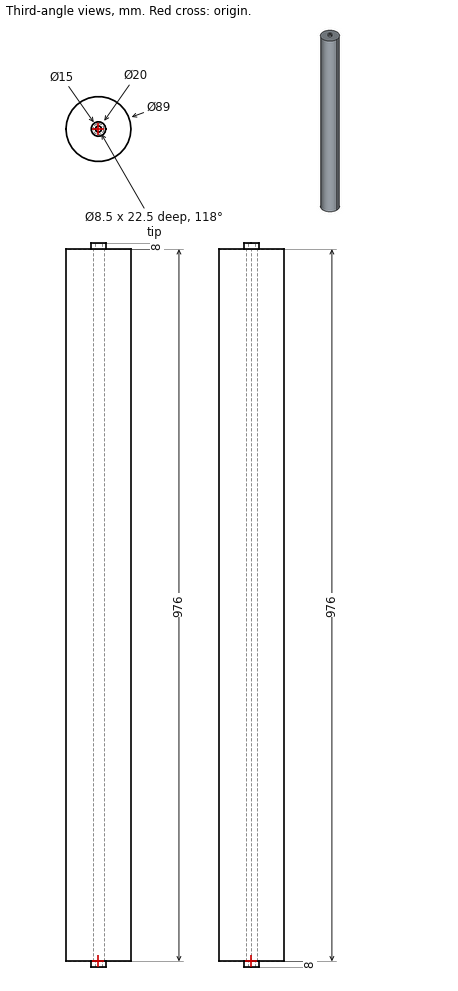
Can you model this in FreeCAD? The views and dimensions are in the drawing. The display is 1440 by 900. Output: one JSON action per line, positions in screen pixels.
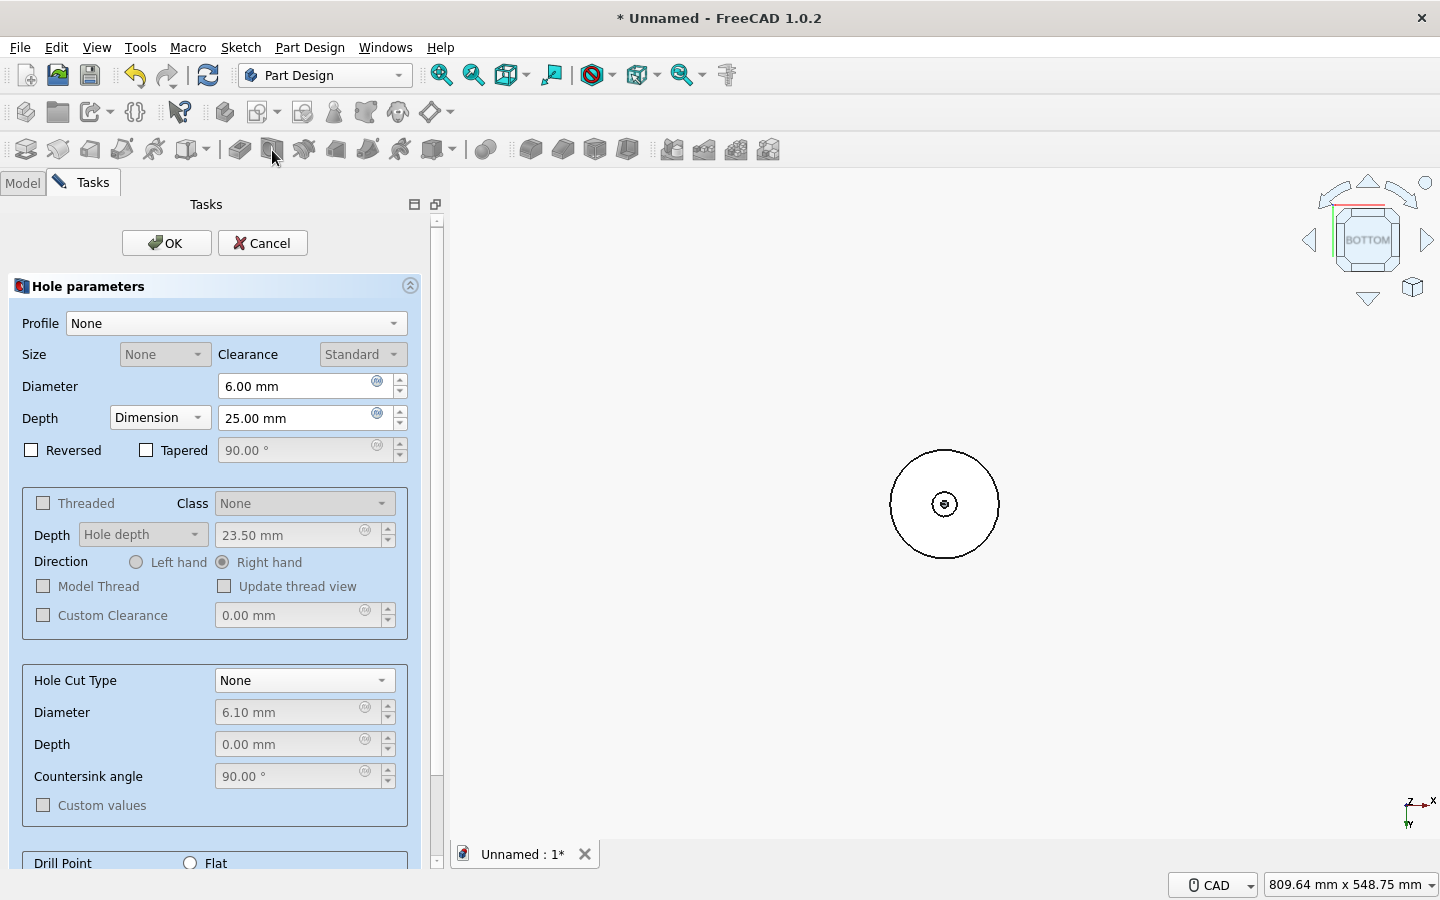
{"action": "triple_click", "coordinate": [305, 386]}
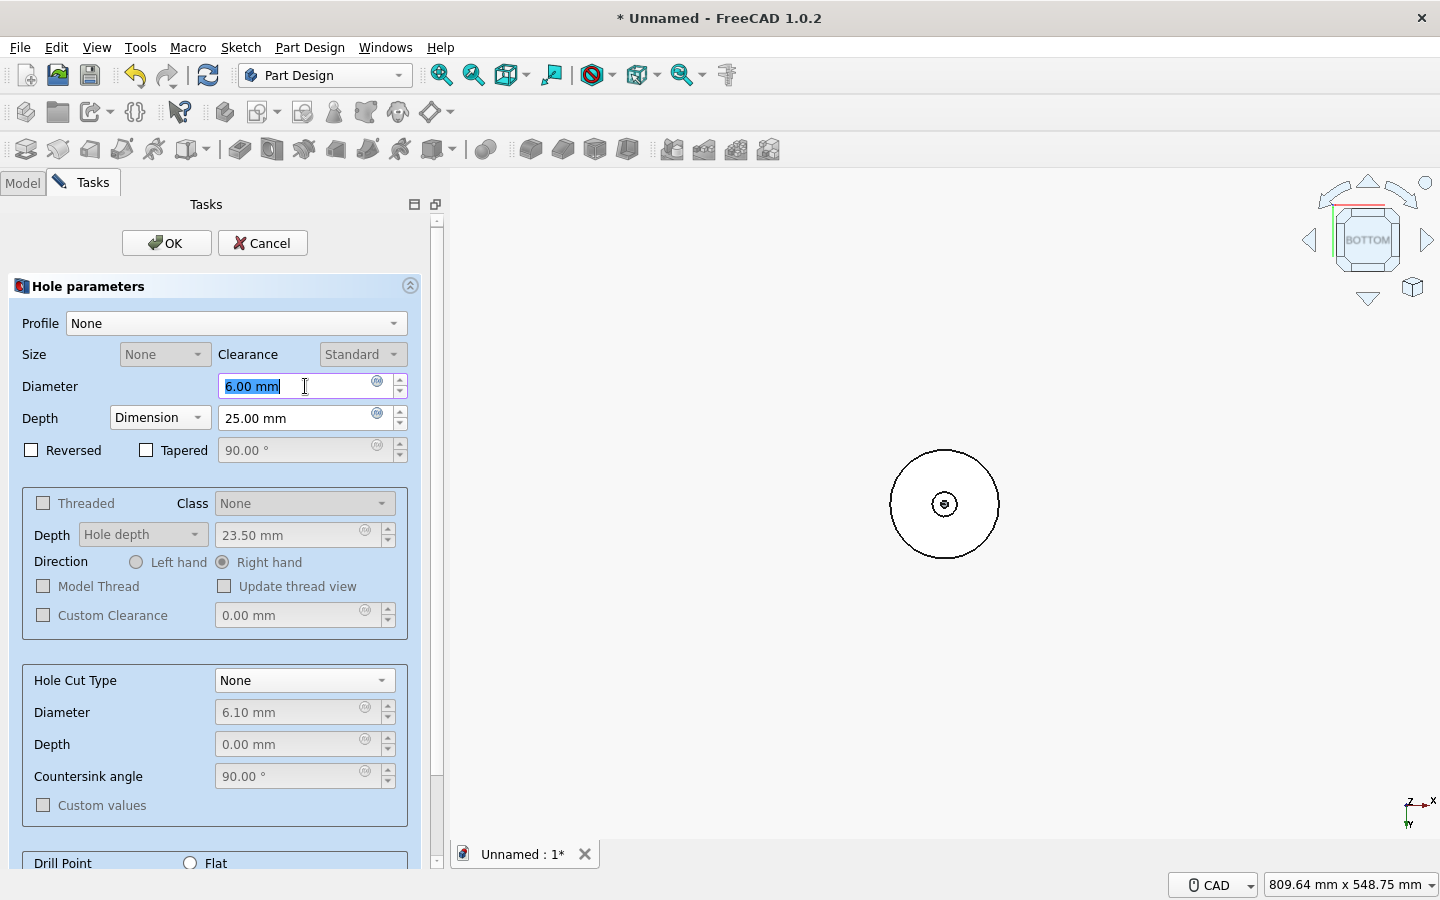
{"action": "type", "text": "8.5"}
{"action": "key", "text": "Tab"}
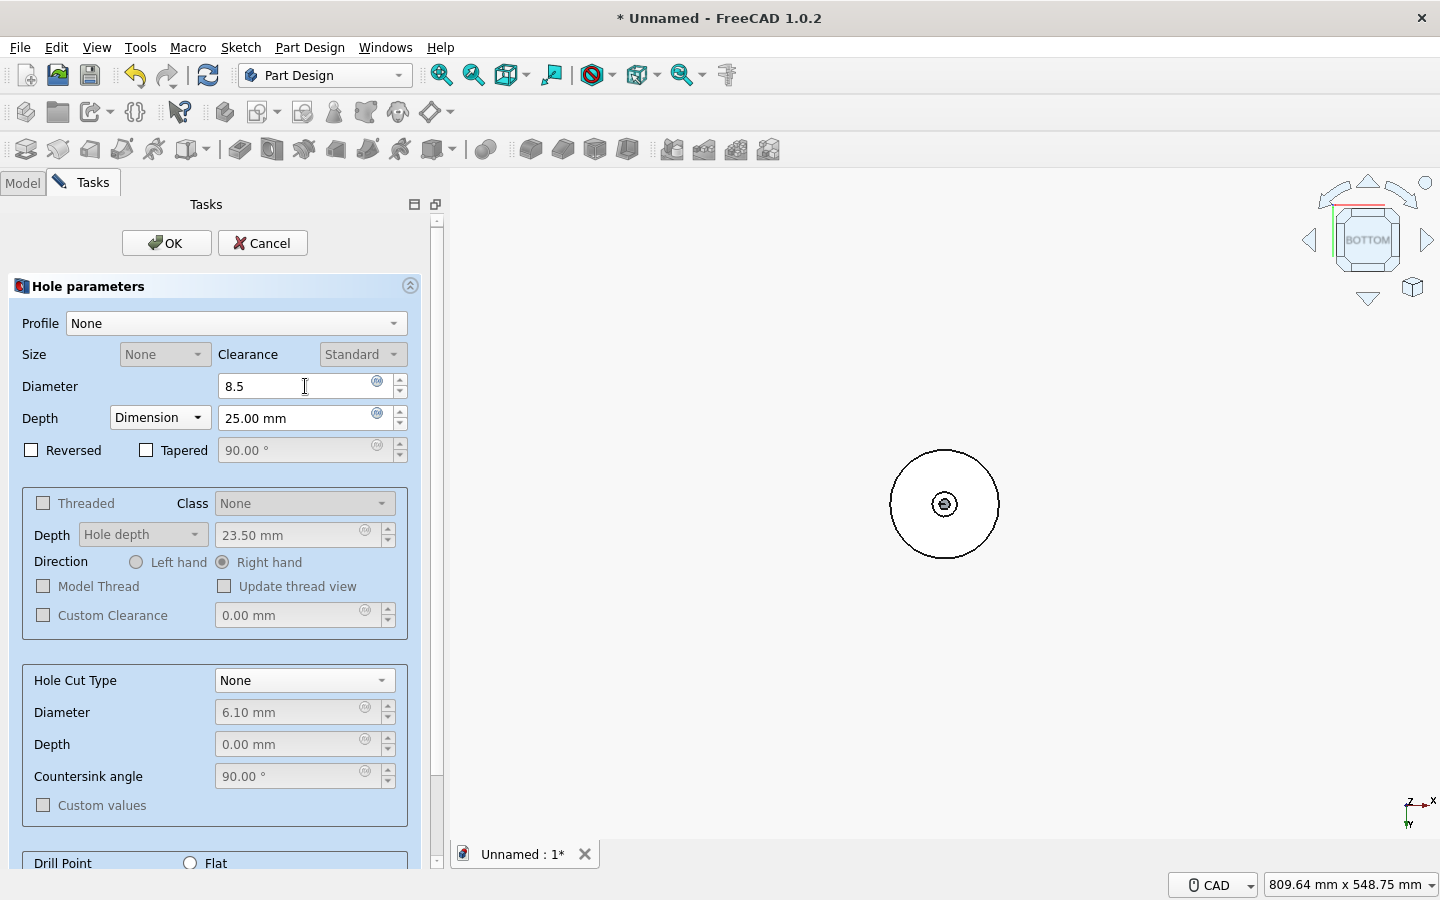
{"action": "triple_click", "coordinate": [305, 418]}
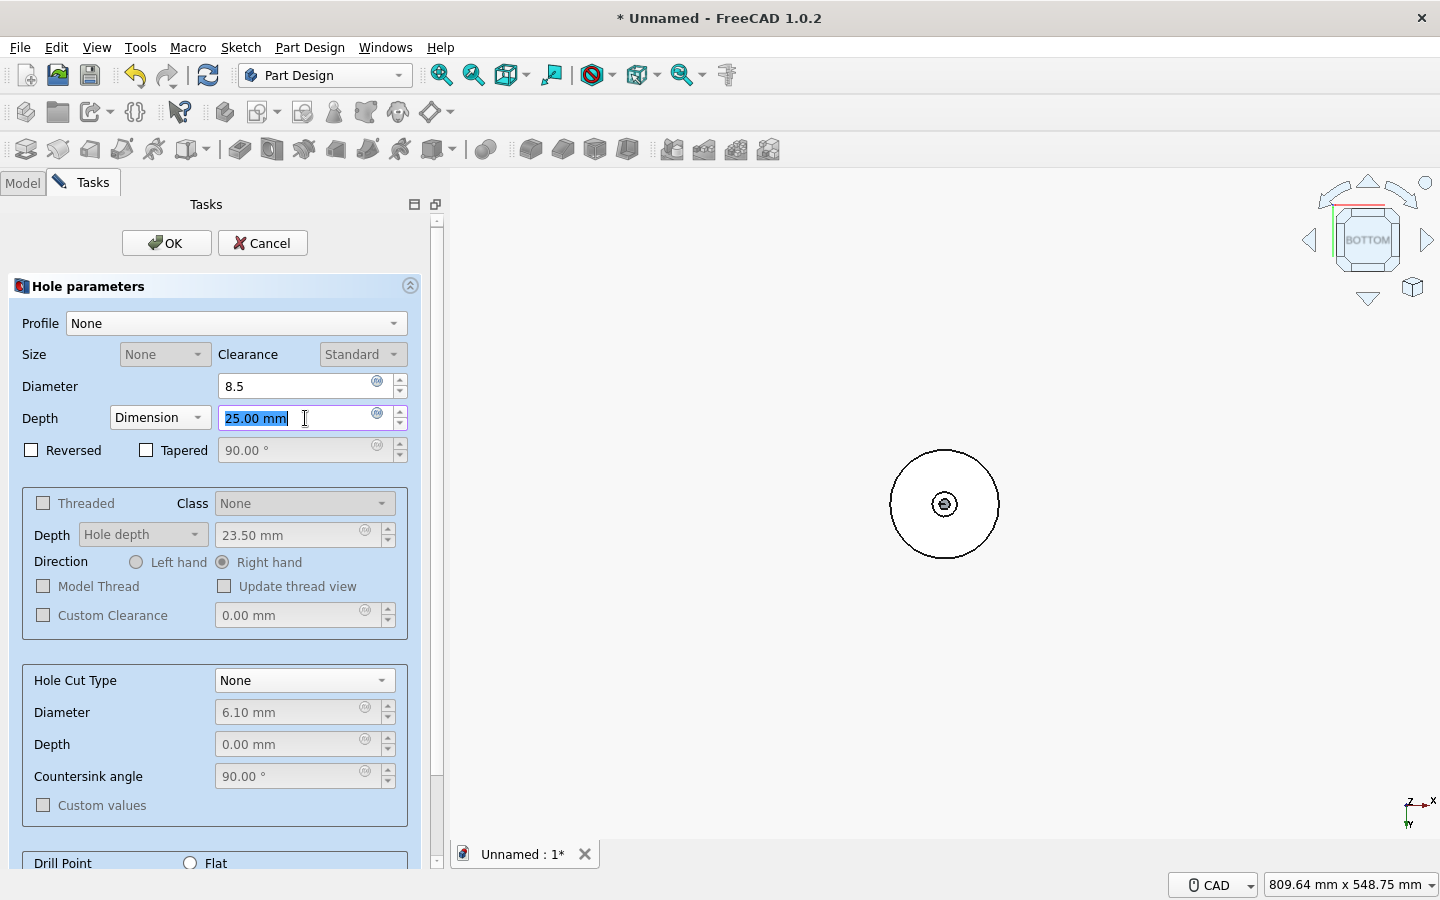
{"action": "type", "text": "22.5"}
{"action": "key", "text": "Tab"}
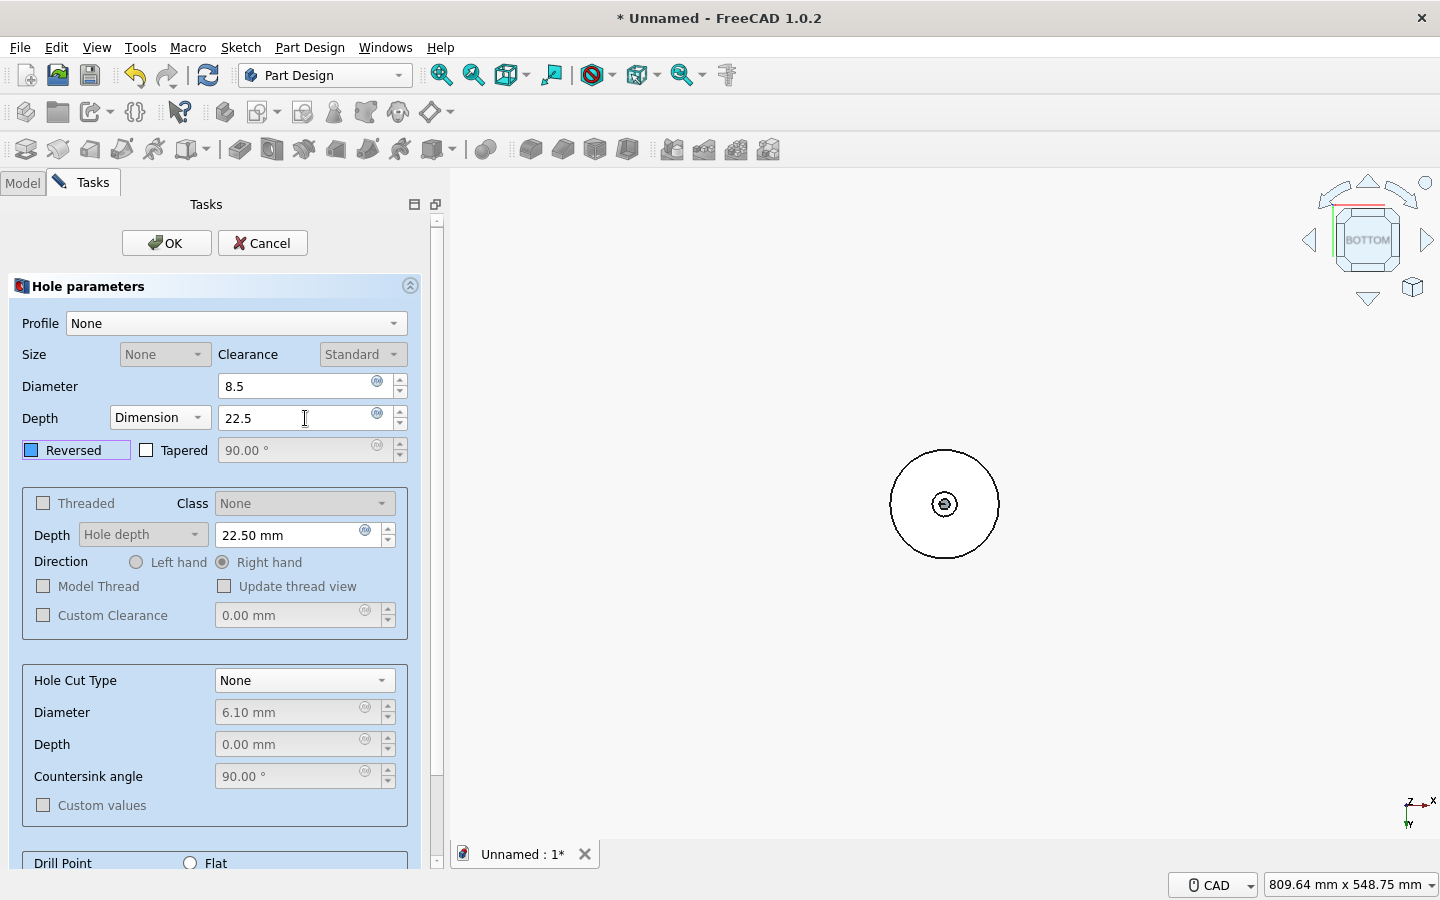
{"action": "left_click", "coordinate": [167, 243]}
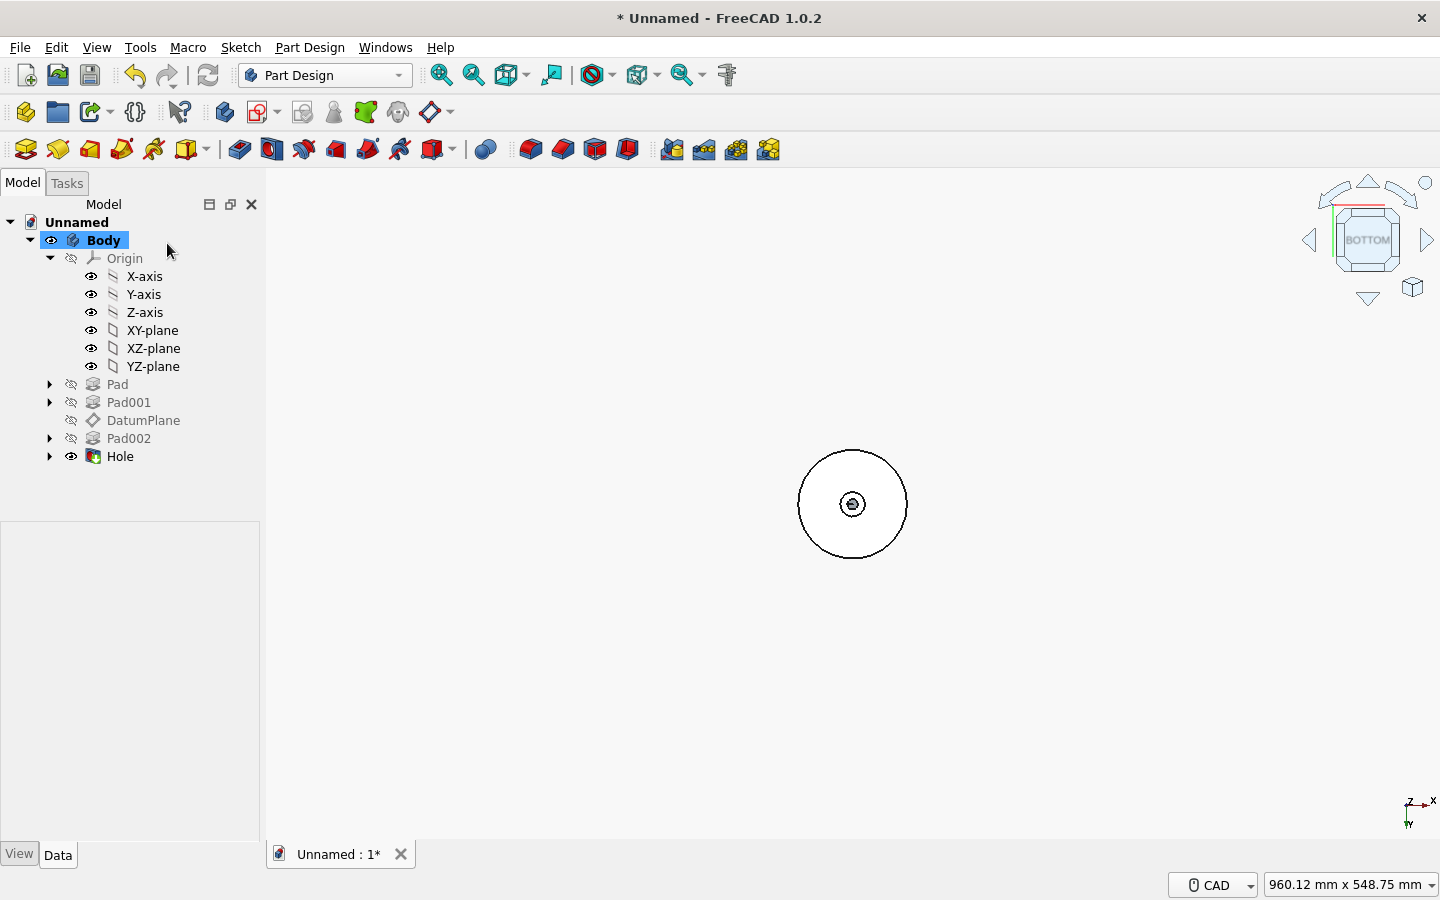
{"action": "left_click", "coordinate": [442, 76]}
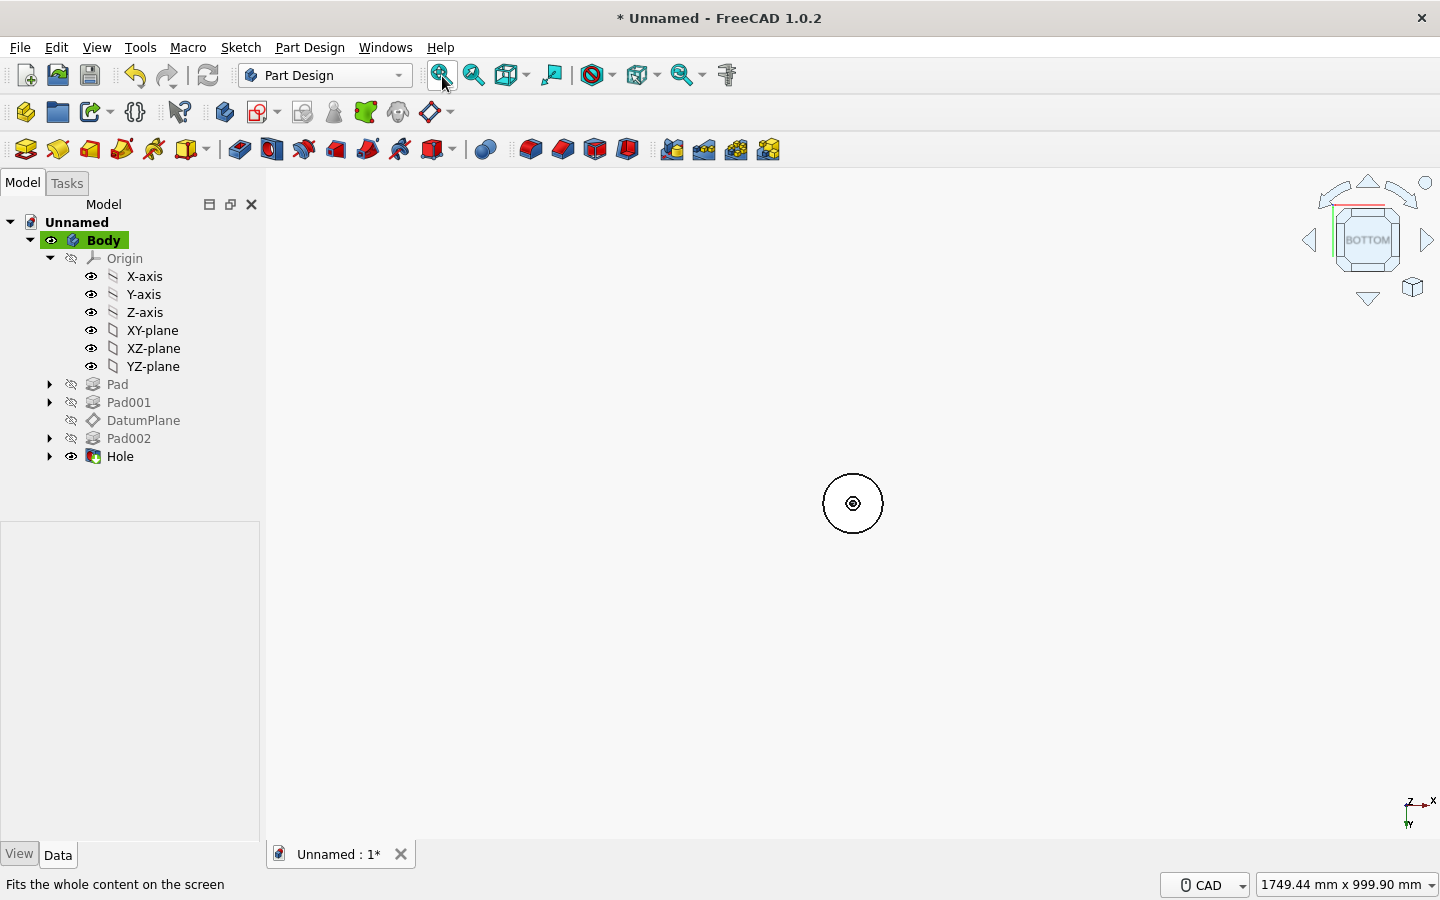
{"action": "key", "text": "0"}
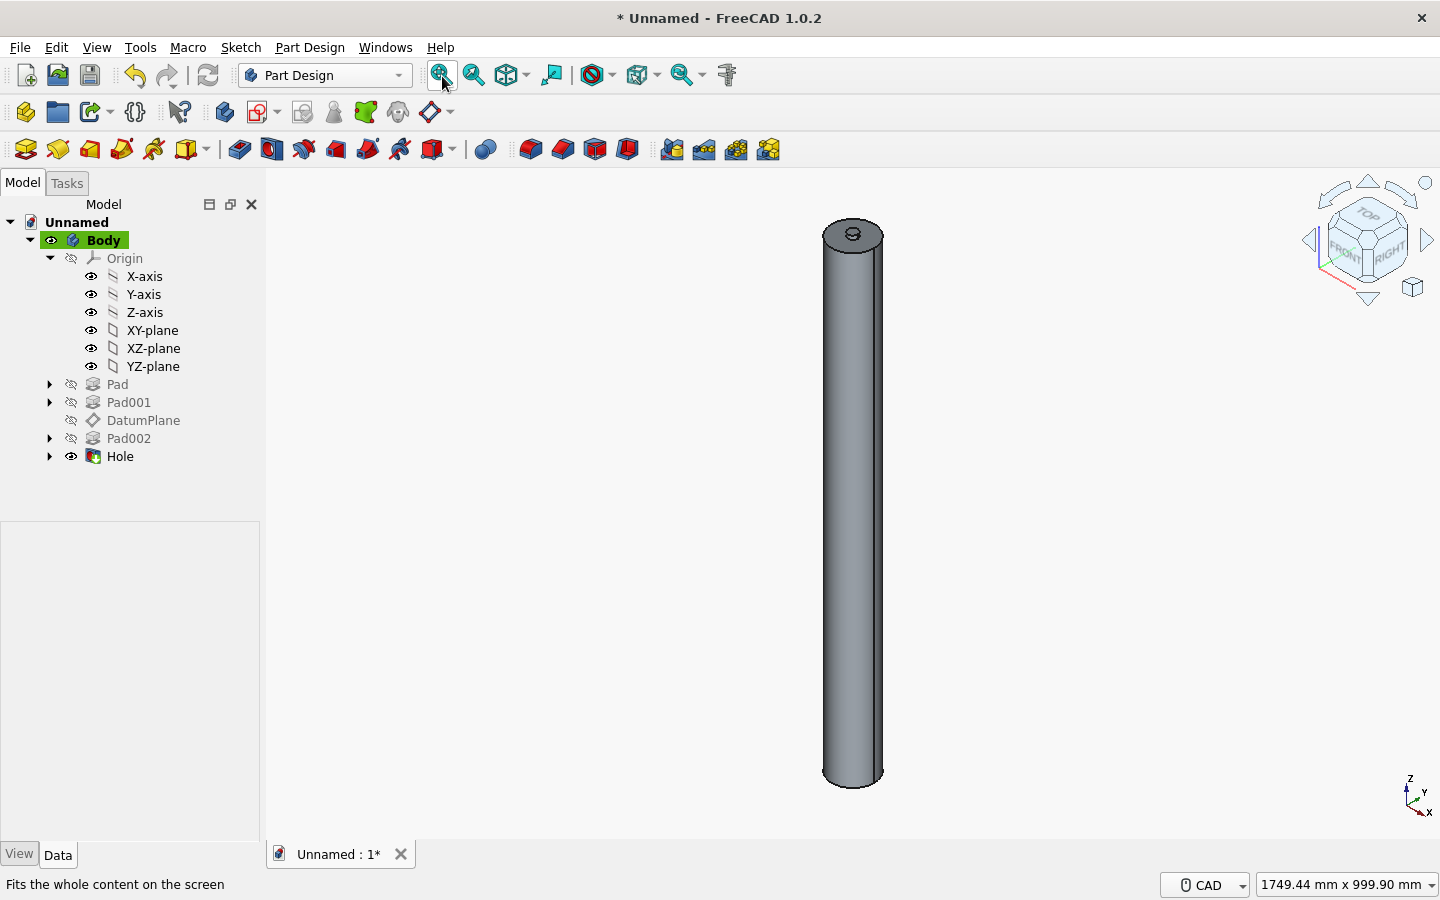
{"action": "scroll", "coordinate": [853, 231], "scroll_direction": "up", "scroll_amount": 3}